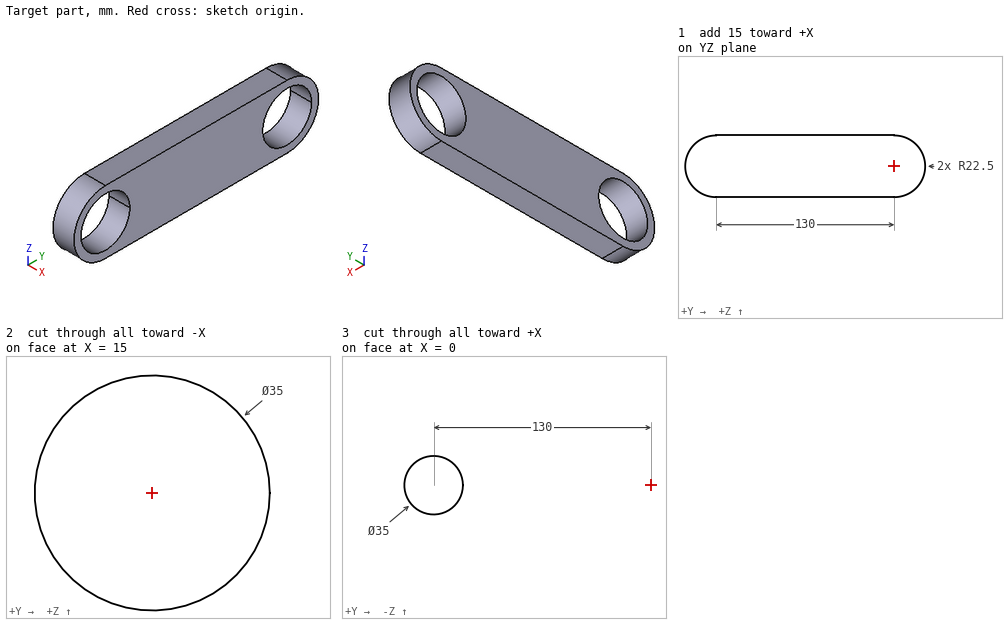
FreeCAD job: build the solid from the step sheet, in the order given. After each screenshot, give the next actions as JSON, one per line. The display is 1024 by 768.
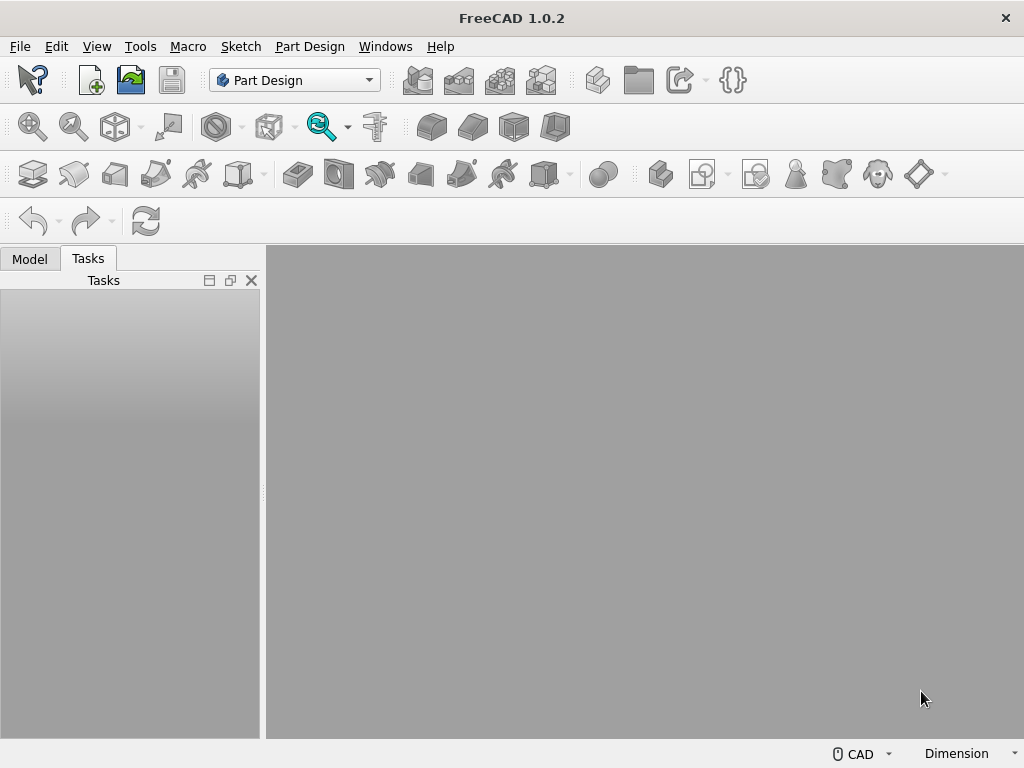
{"action": "left_click", "coordinate": [90, 80]}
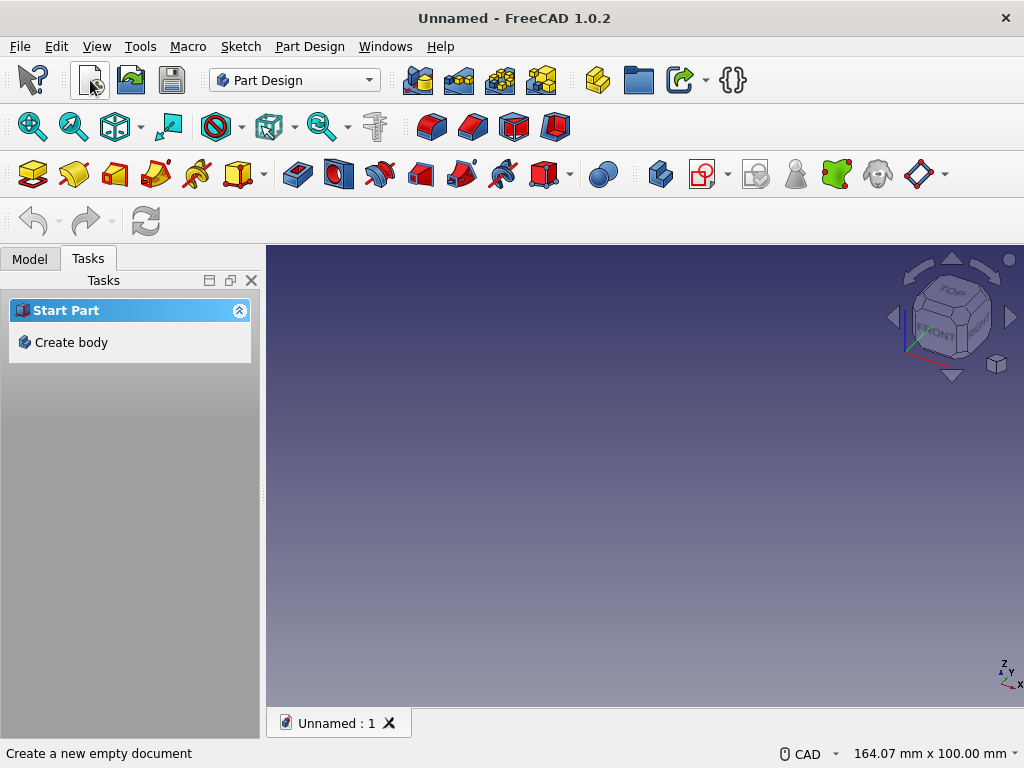
{"action": "left_click", "coordinate": [702, 174]}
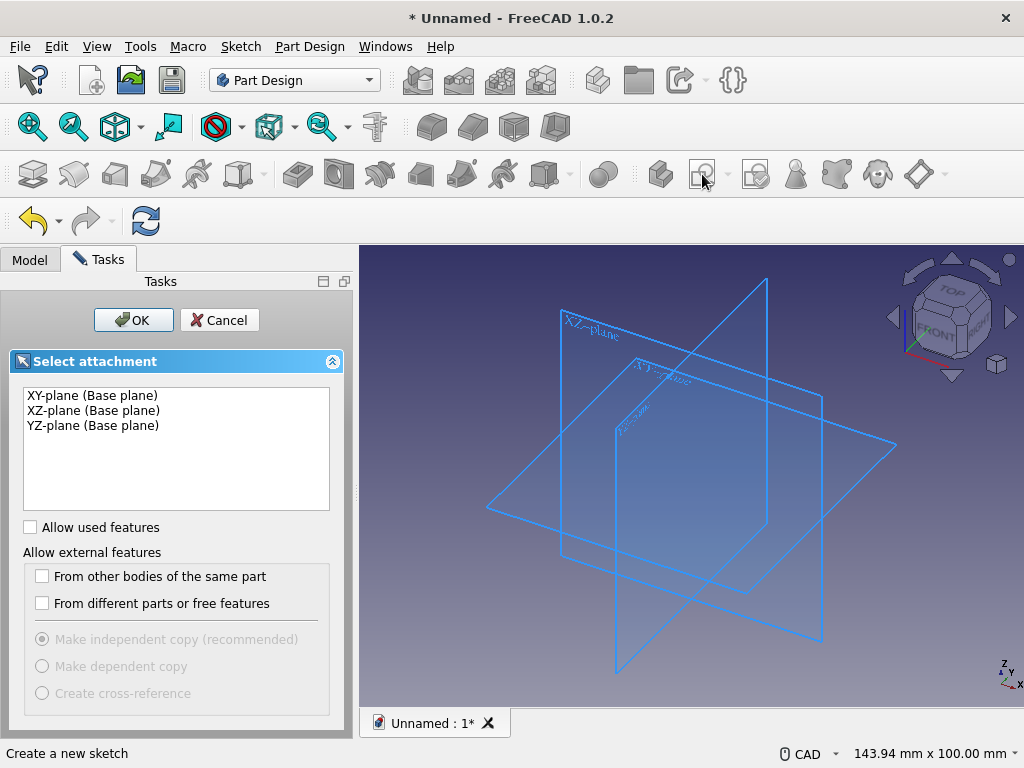
{"action": "left_click", "coordinate": [84, 426]}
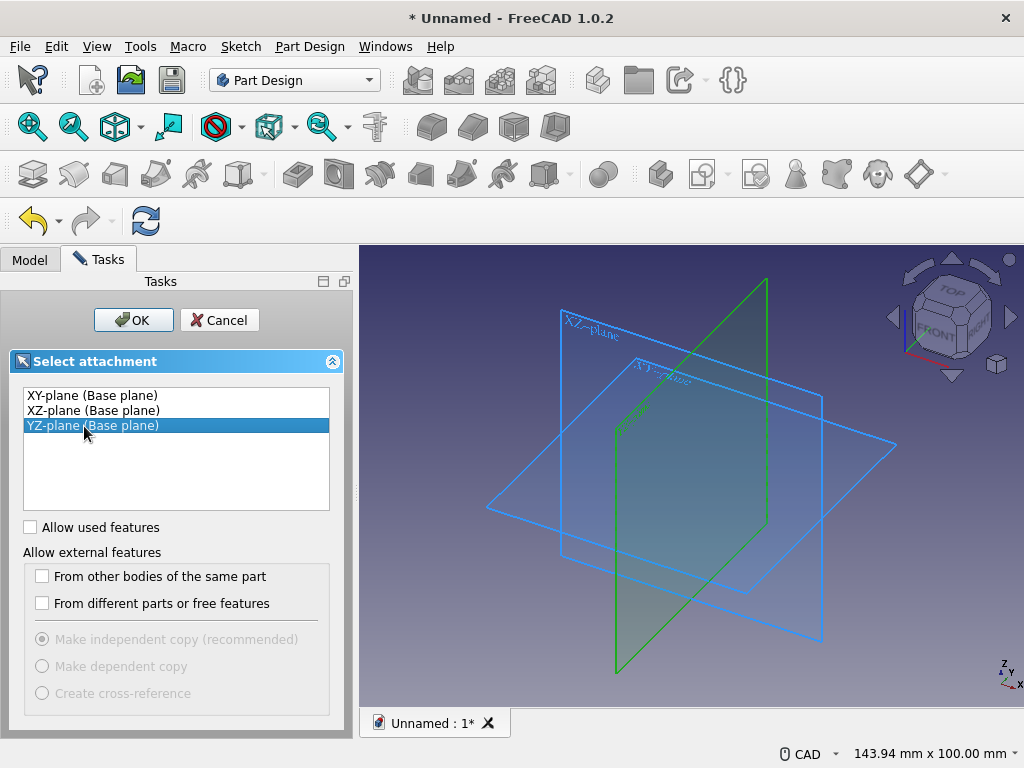
{"action": "left_click", "coordinate": [134, 320]}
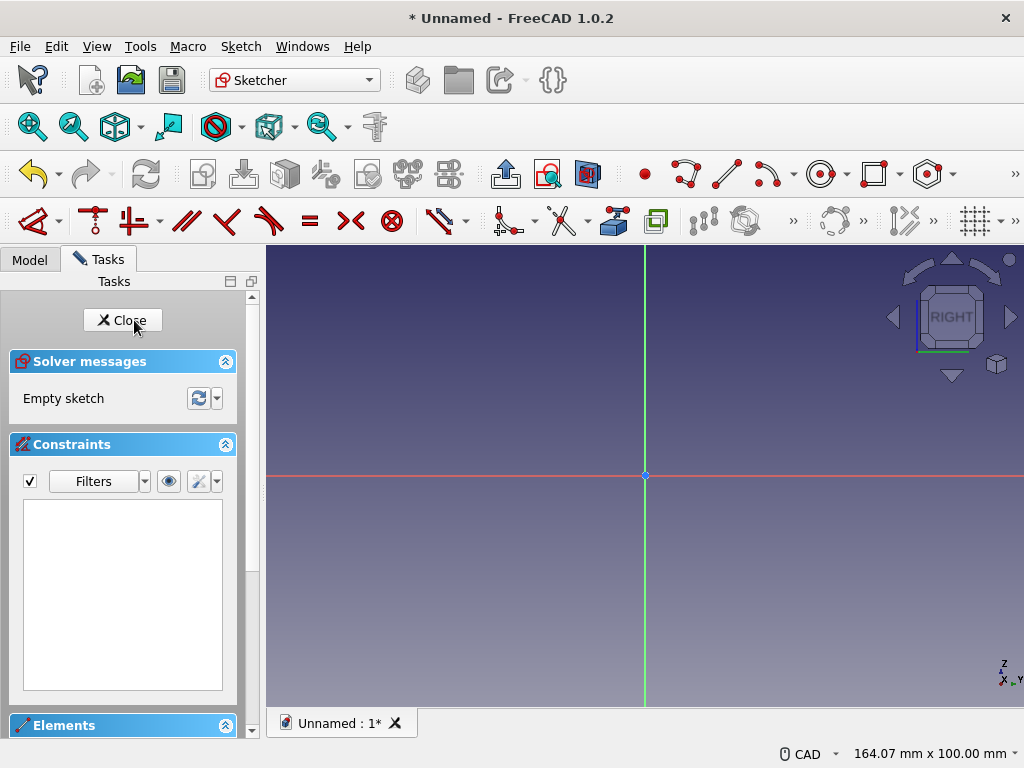
{"action": "scroll", "coordinate": [766, 476], "scroll_direction": "down", "scroll_amount": 4}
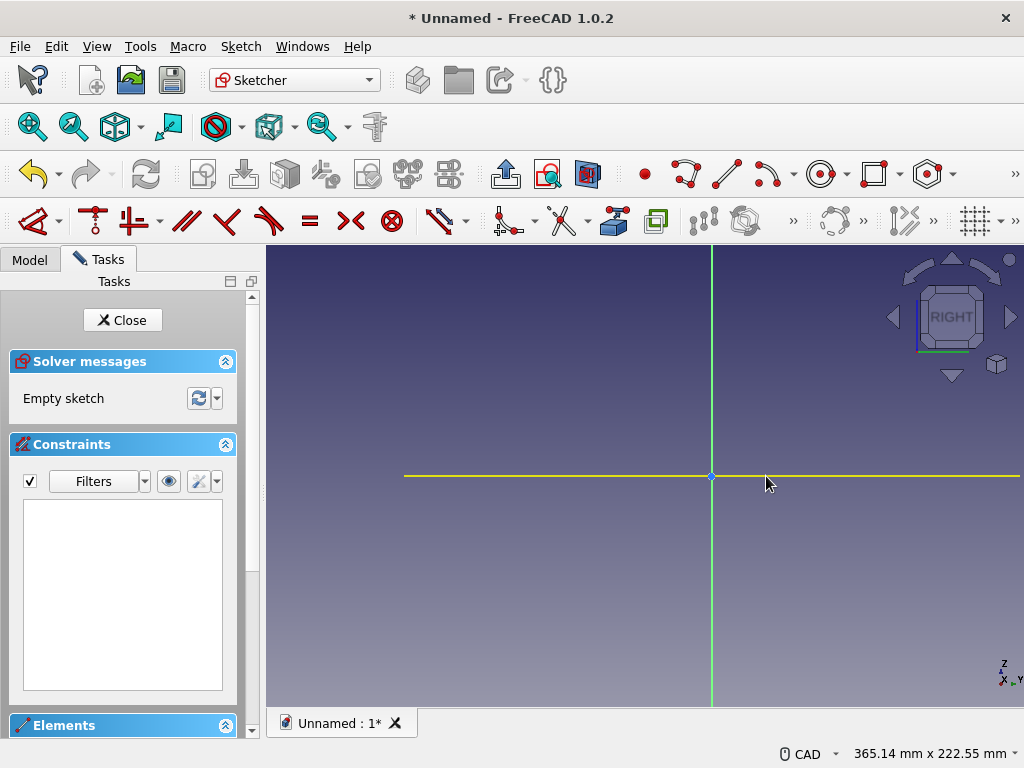
{"action": "key", "text": "g s"}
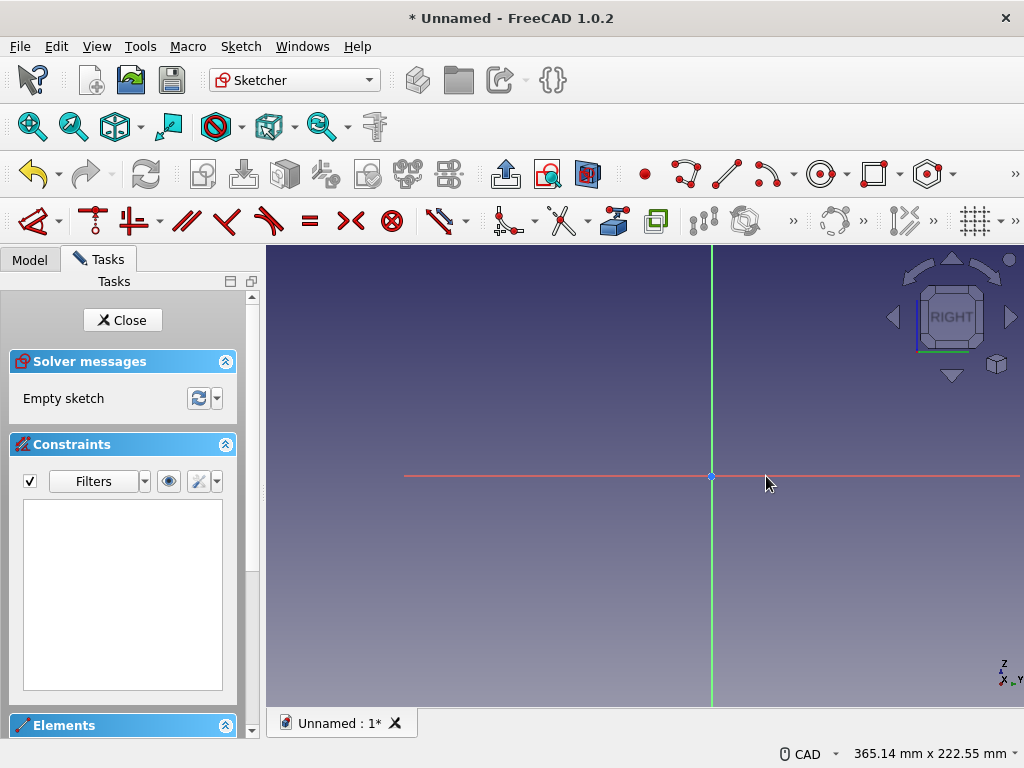
{"action": "left_click", "coordinate": [712, 476]}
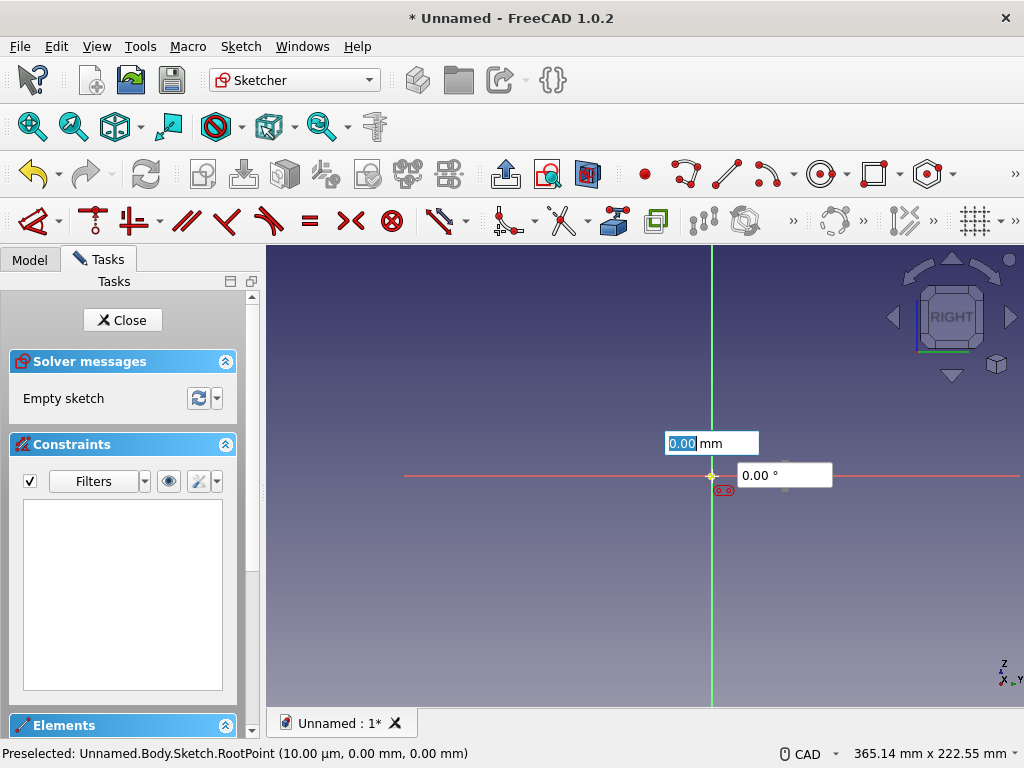
{"action": "left_click", "coordinate": [442, 467]}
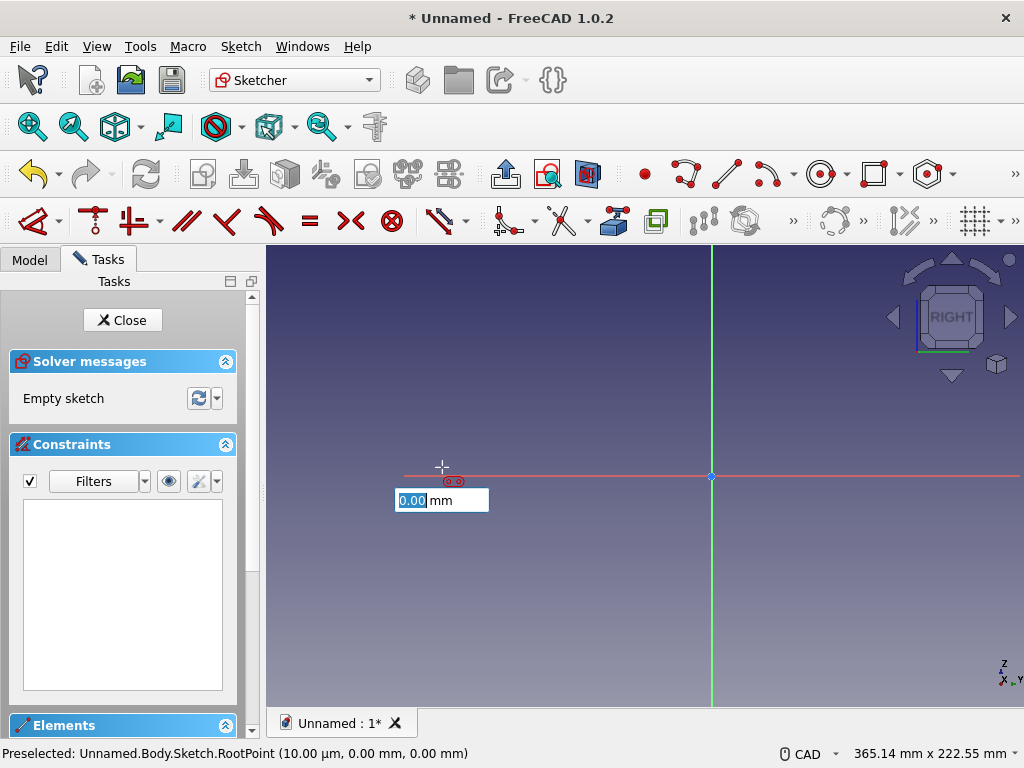
{"action": "left_click", "coordinate": [577, 523]}
{"action": "key", "text": "Escape"}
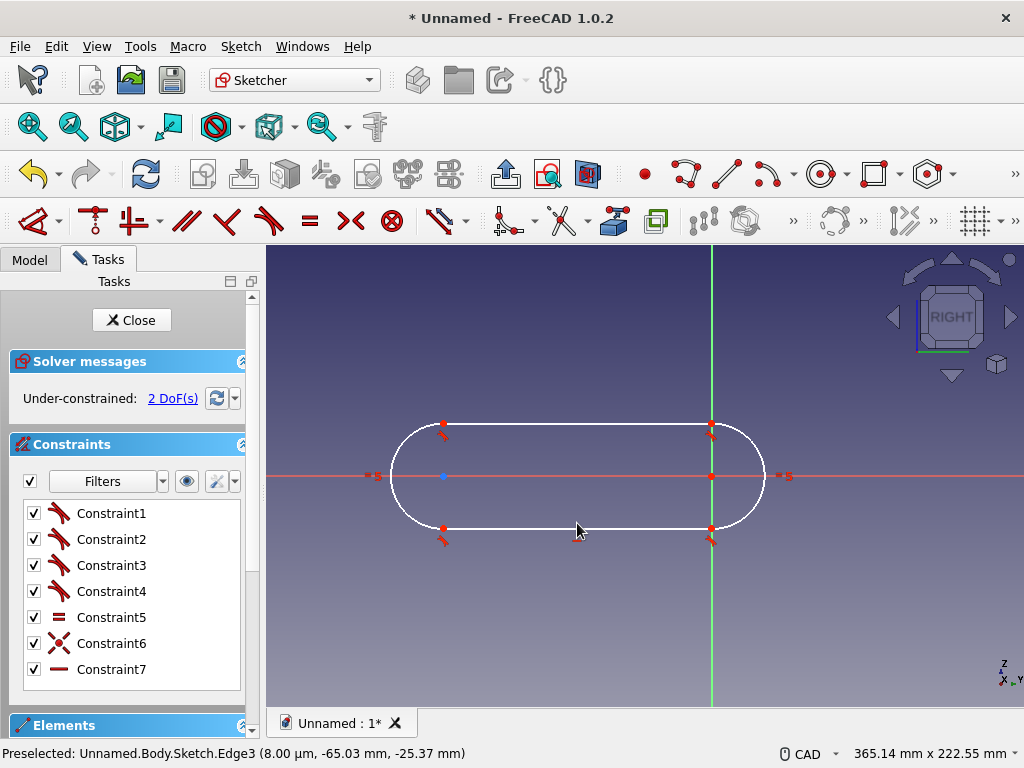
{"action": "left_click", "coordinate": [755, 507]}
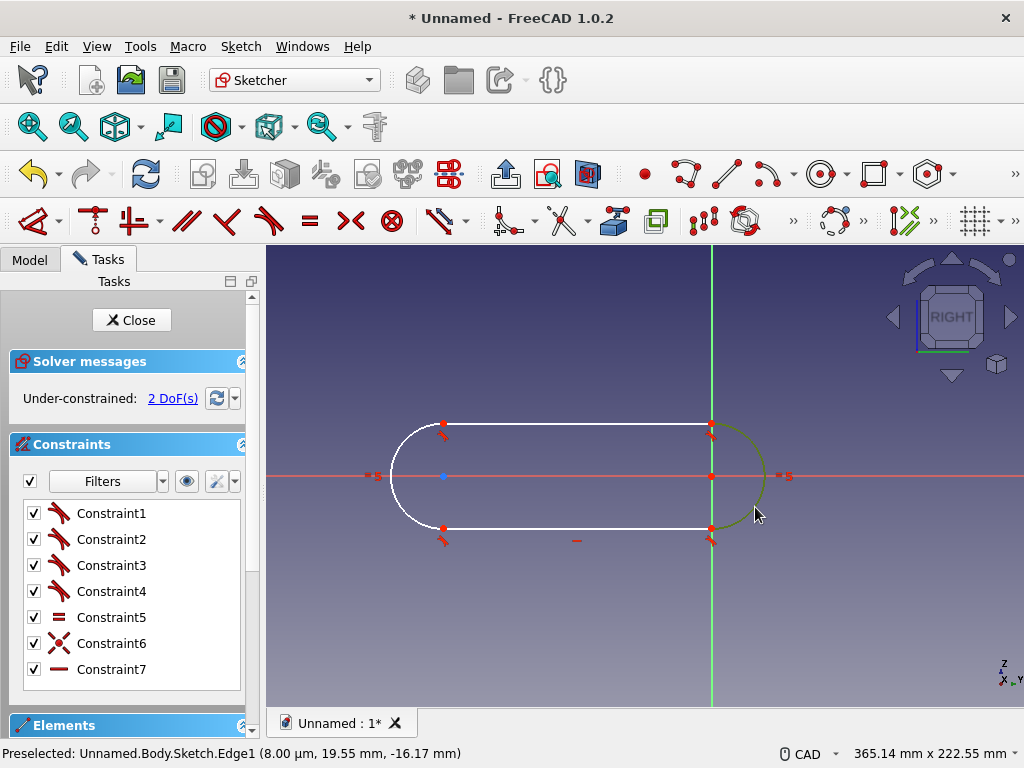
{"action": "left_click", "coordinate": [58, 222]}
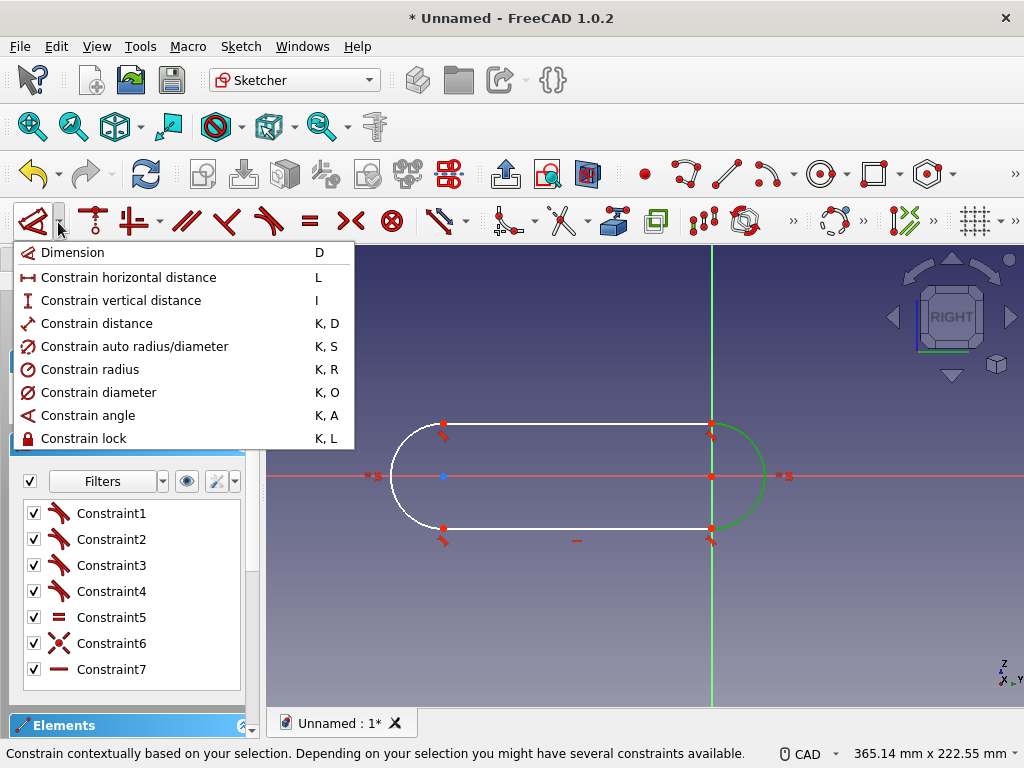
{"action": "left_click", "coordinate": [184, 370]}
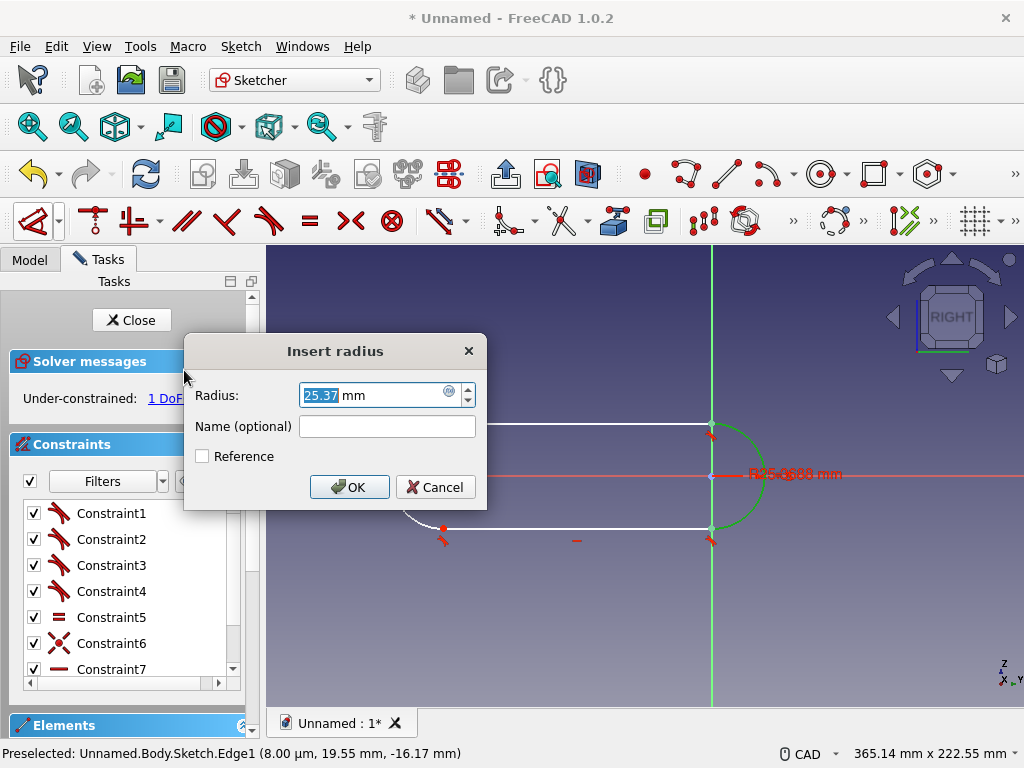
{"action": "type", "text": "22.5"}
{"action": "key", "text": "Return"}